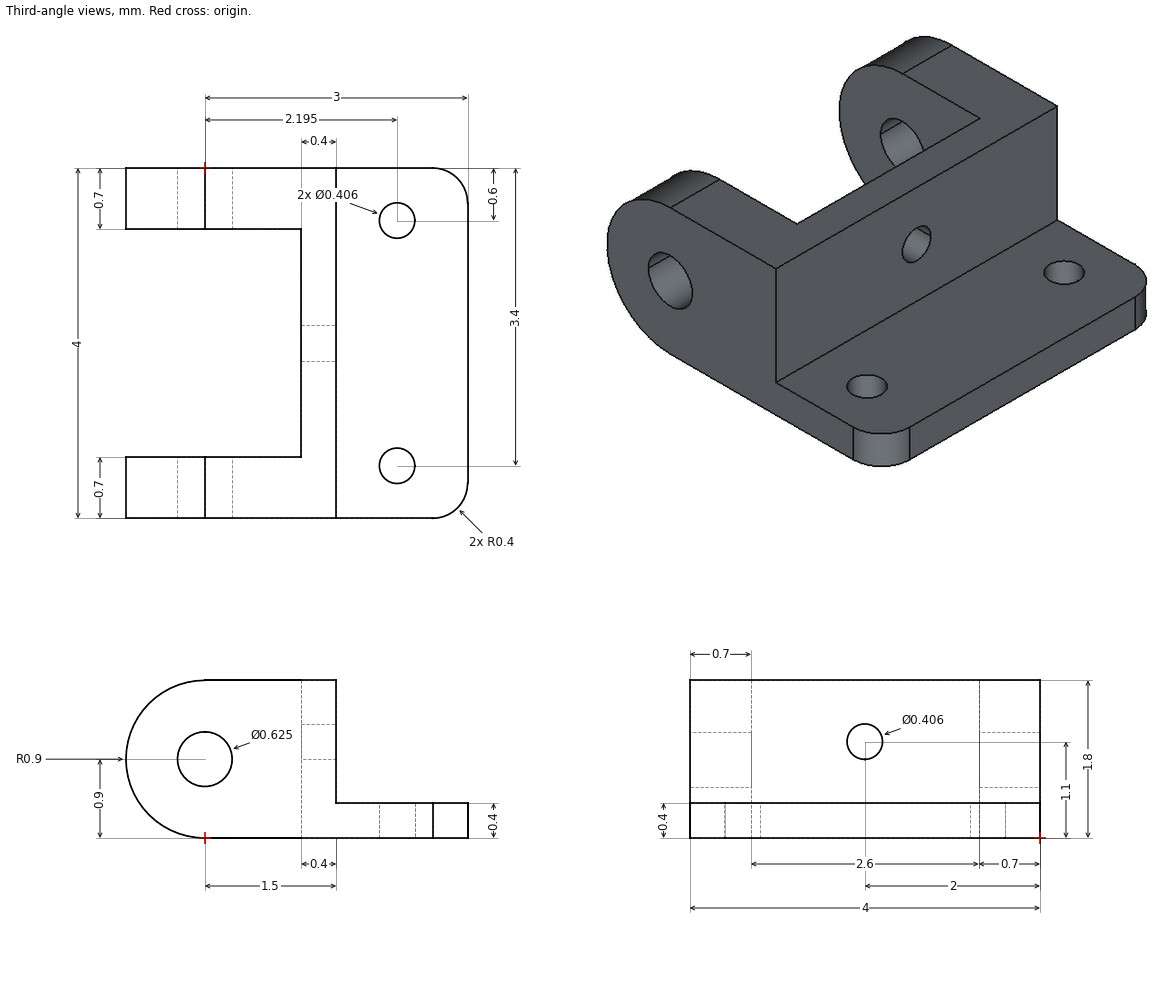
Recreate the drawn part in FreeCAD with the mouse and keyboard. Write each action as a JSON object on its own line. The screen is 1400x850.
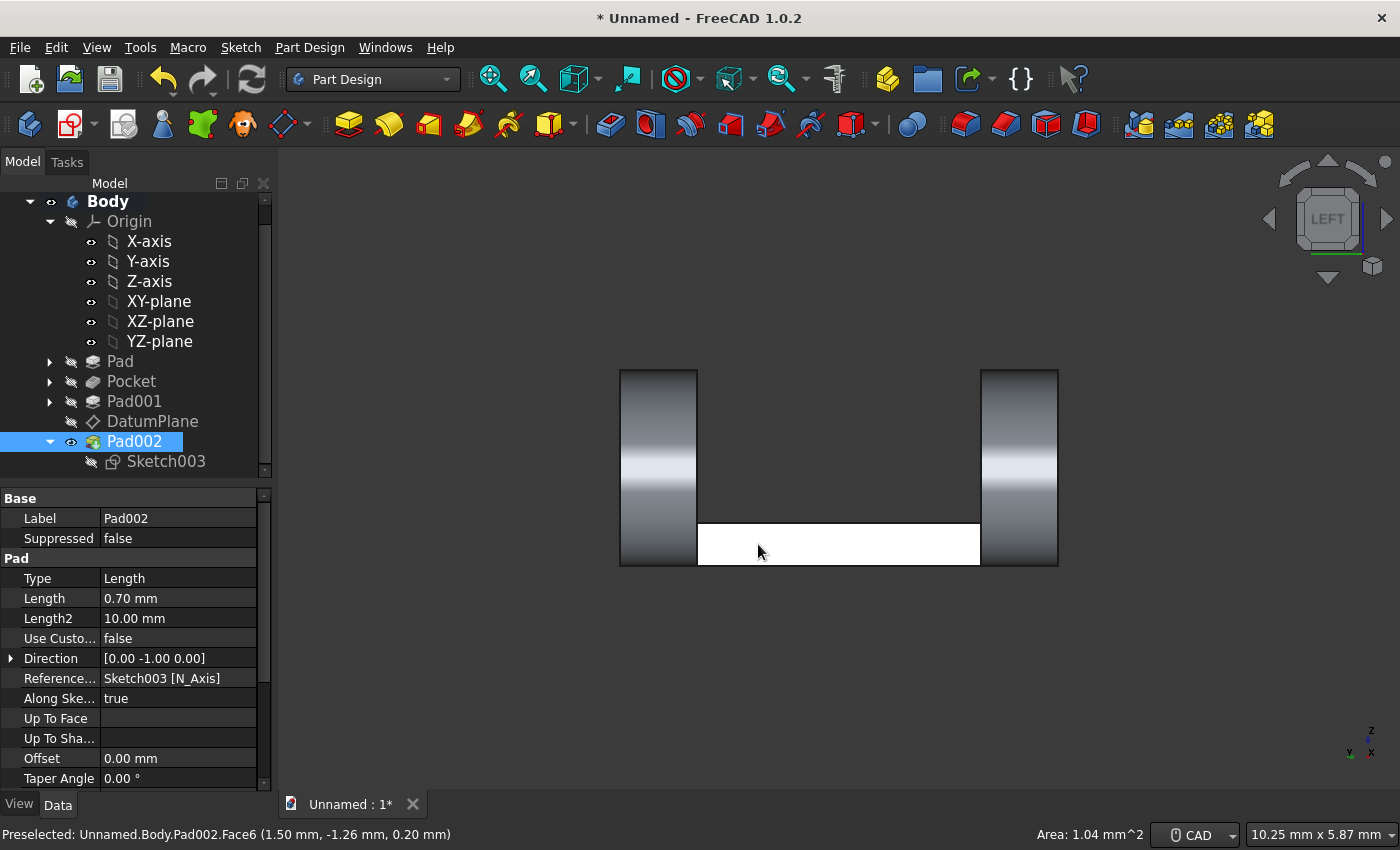
{"action": "left_click", "coordinate": [70, 124]}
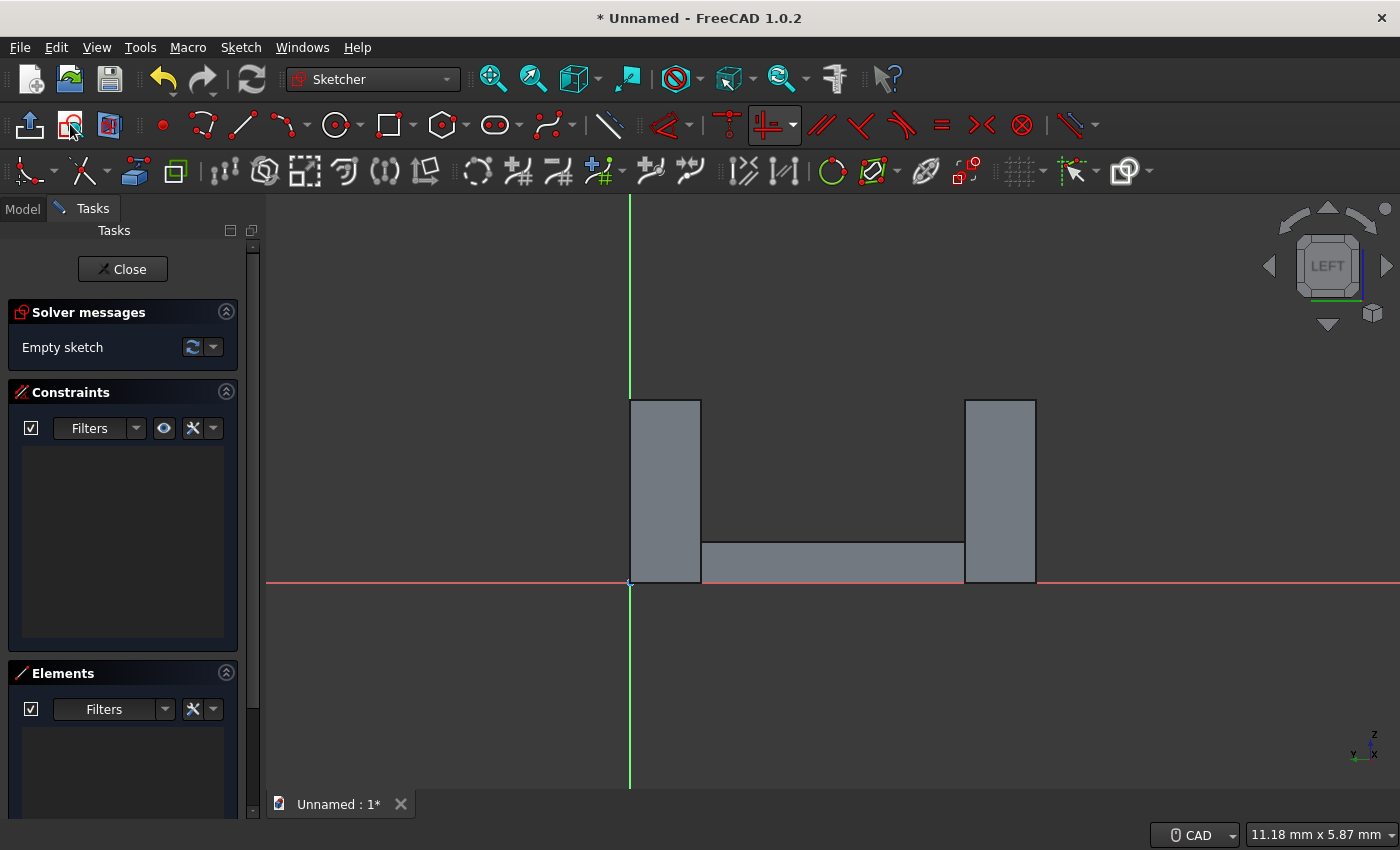
{"action": "scroll", "coordinate": [838, 491], "scroll_direction": "up", "scroll_amount": 3}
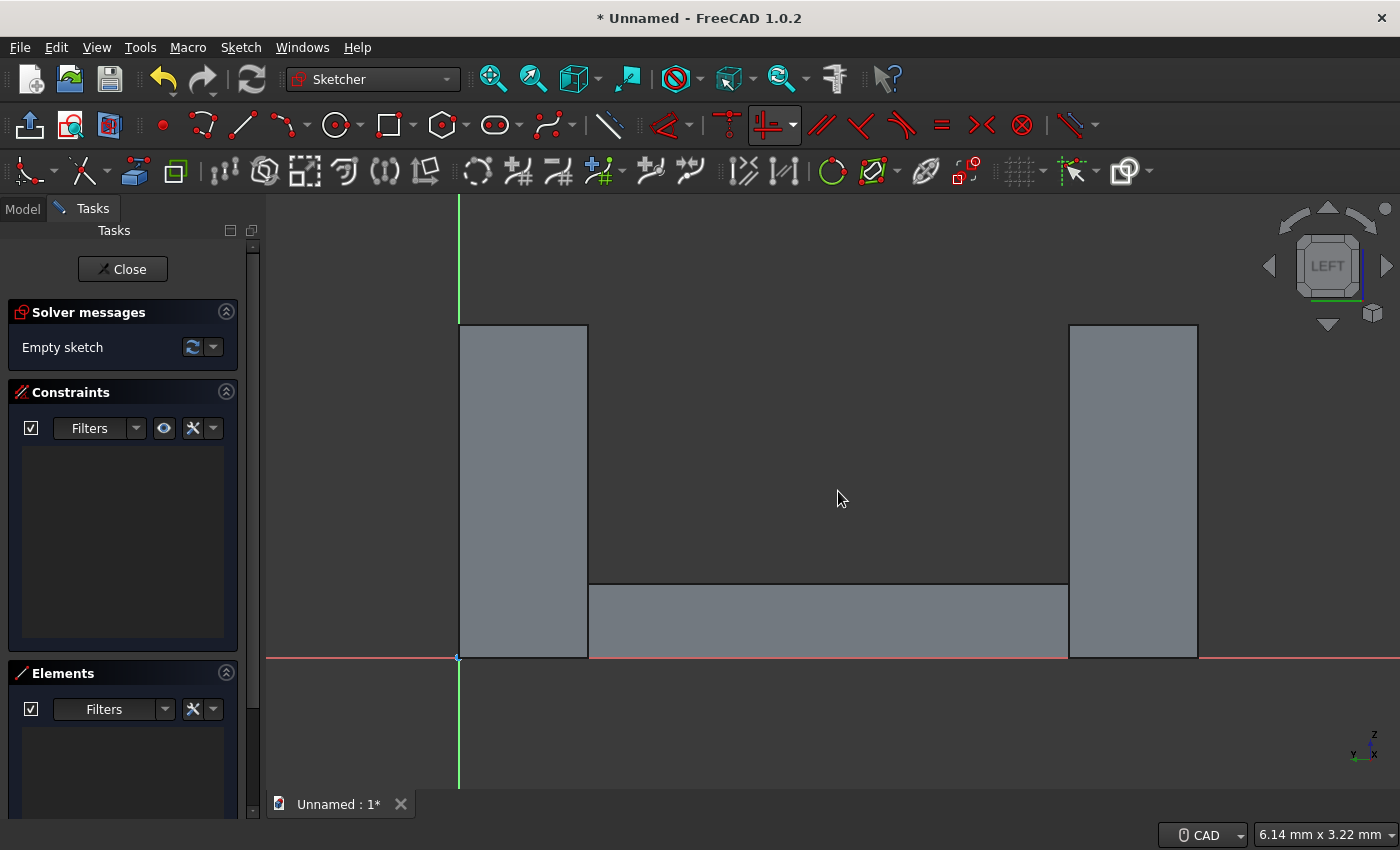
{"action": "key", "text": "g r"}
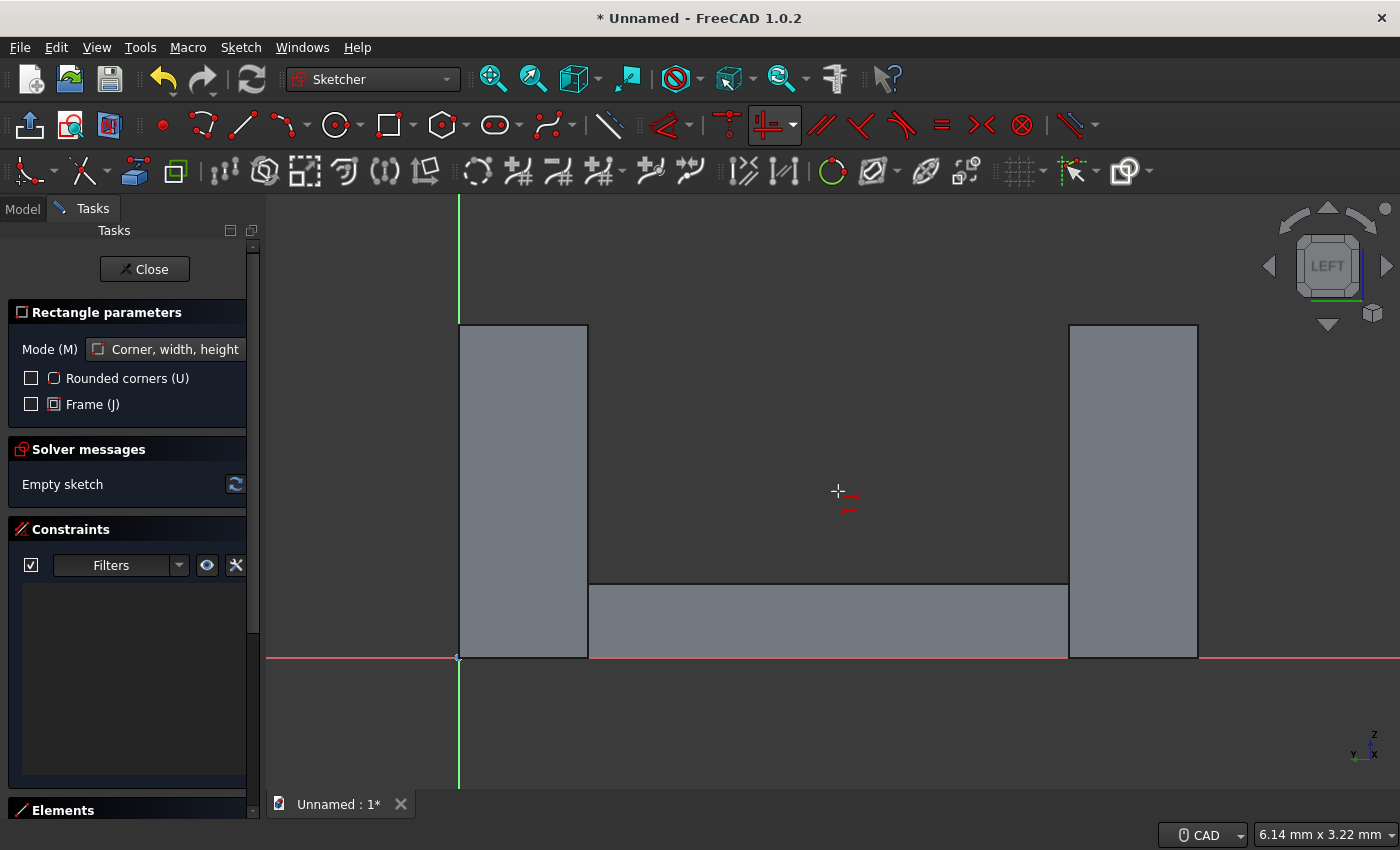
{"action": "left_click", "coordinate": [588, 325]}
{"action": "left_click", "coordinate": [1069, 658]}
{"action": "key", "text": "Escape"}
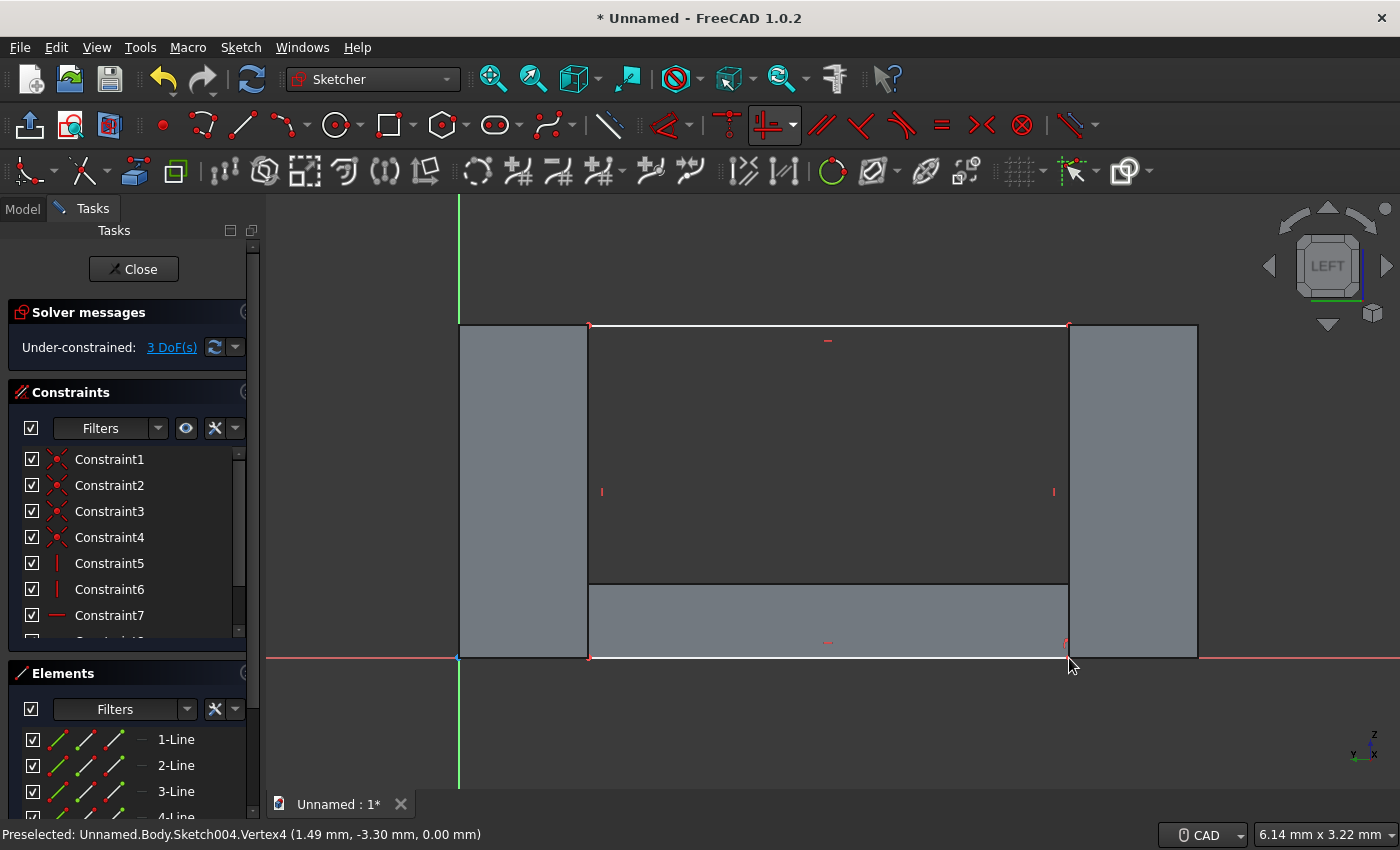
{"action": "key", "text": "d"}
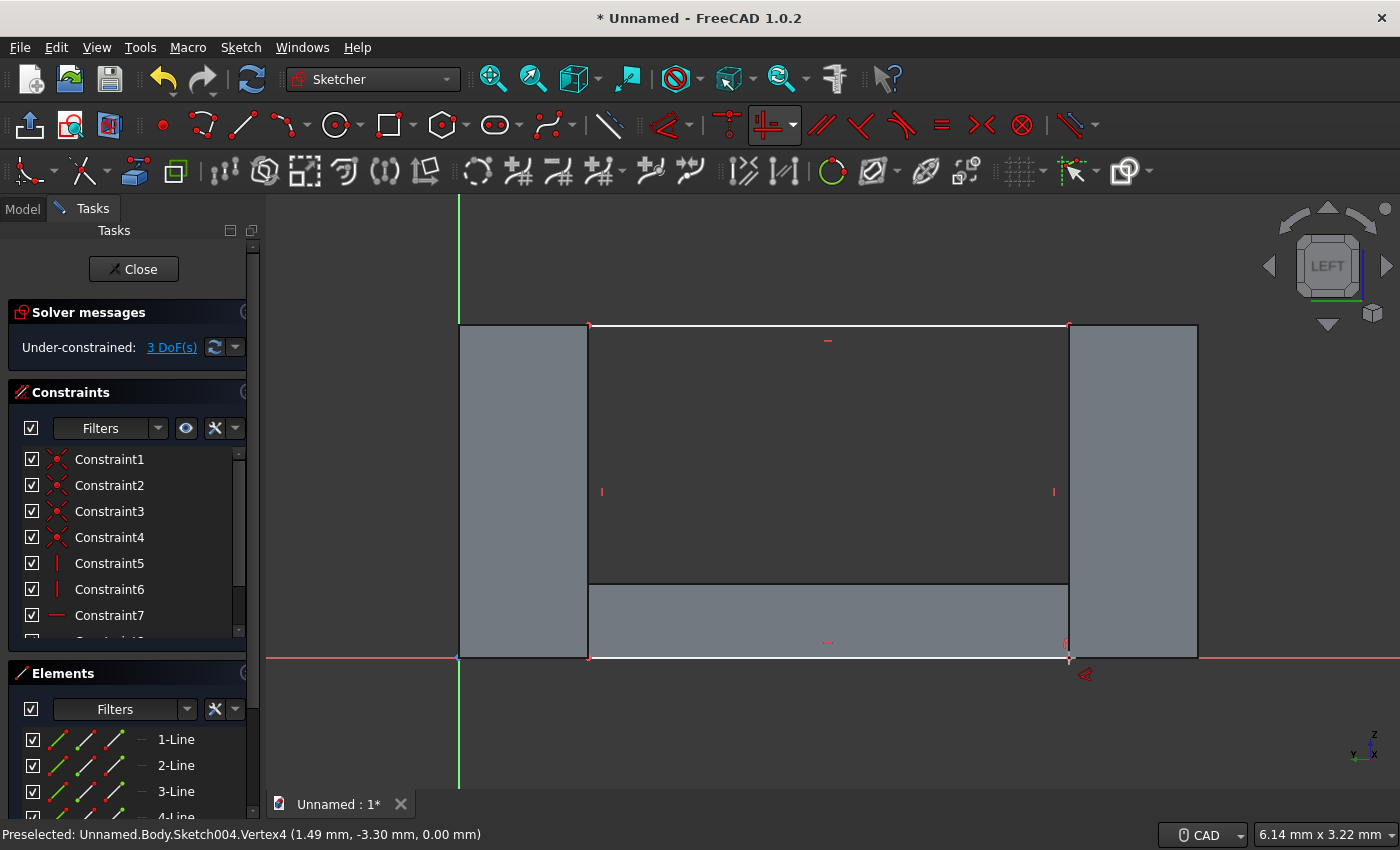
{"action": "left_click", "coordinate": [588, 426]}
{"action": "left_click", "coordinate": [554, 492]}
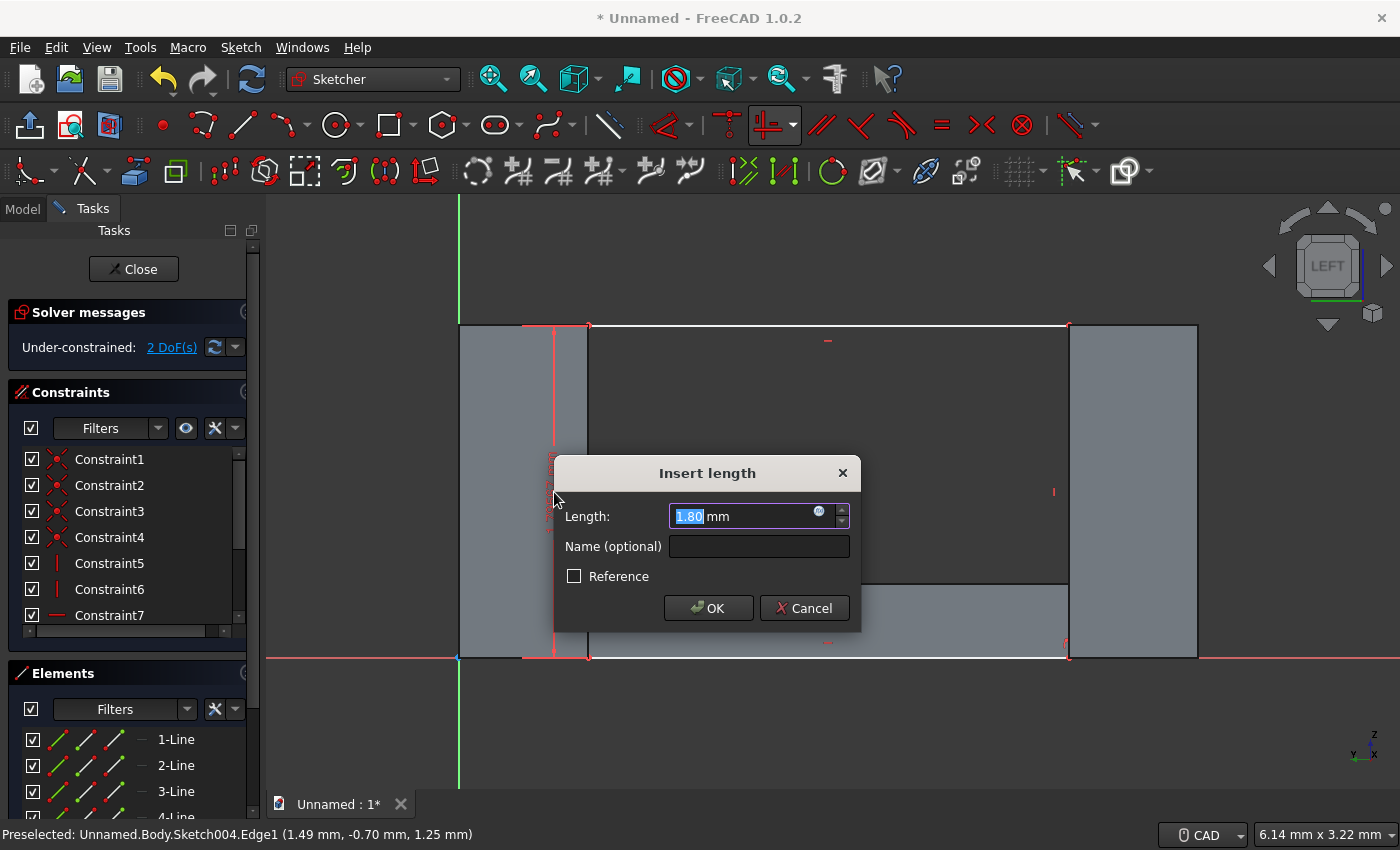
{"action": "type", "text": "1.8"}
{"action": "key", "text": "Return"}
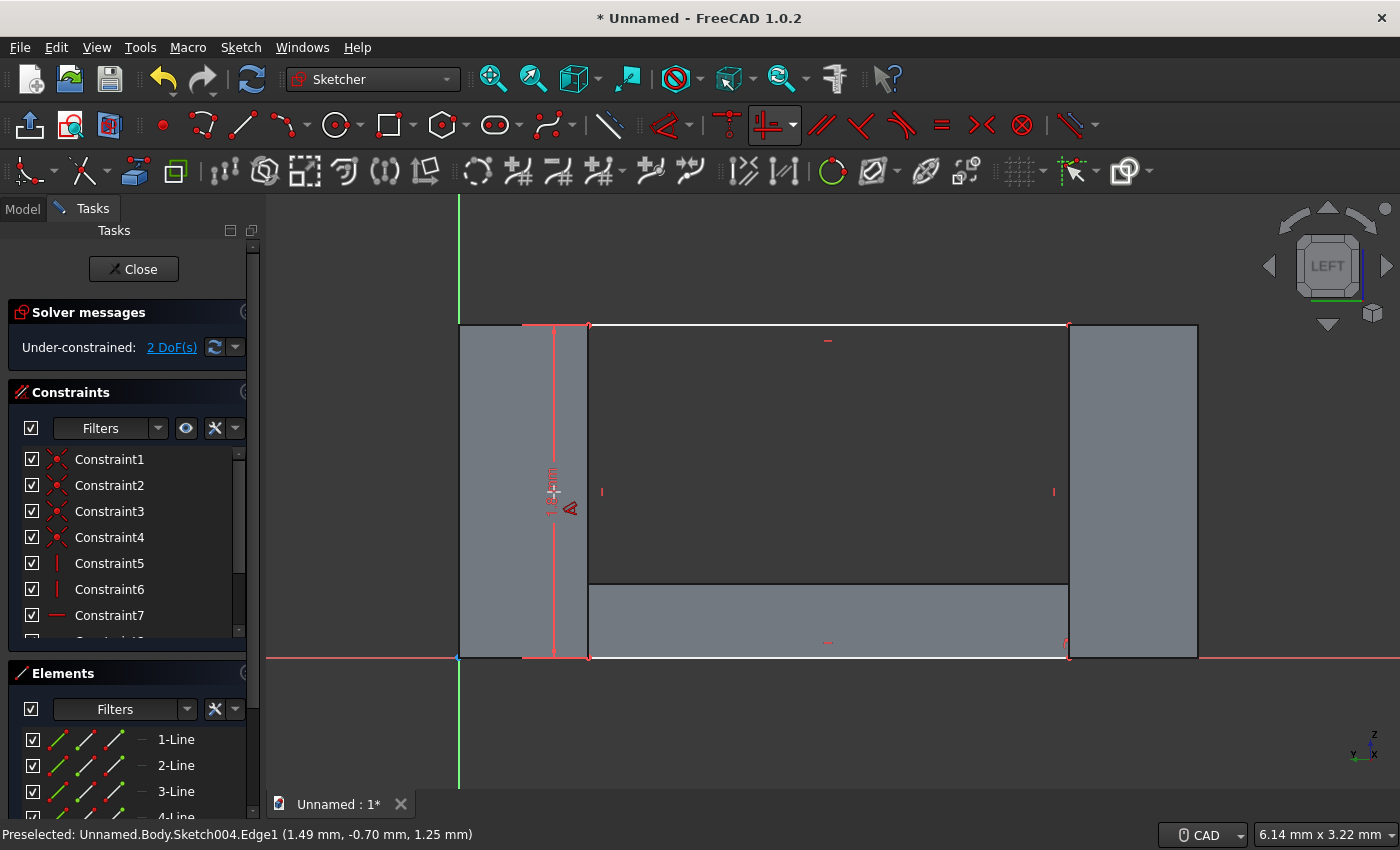
{"action": "left_click", "coordinate": [732, 658]}
{"action": "left_click", "coordinate": [829, 692]}